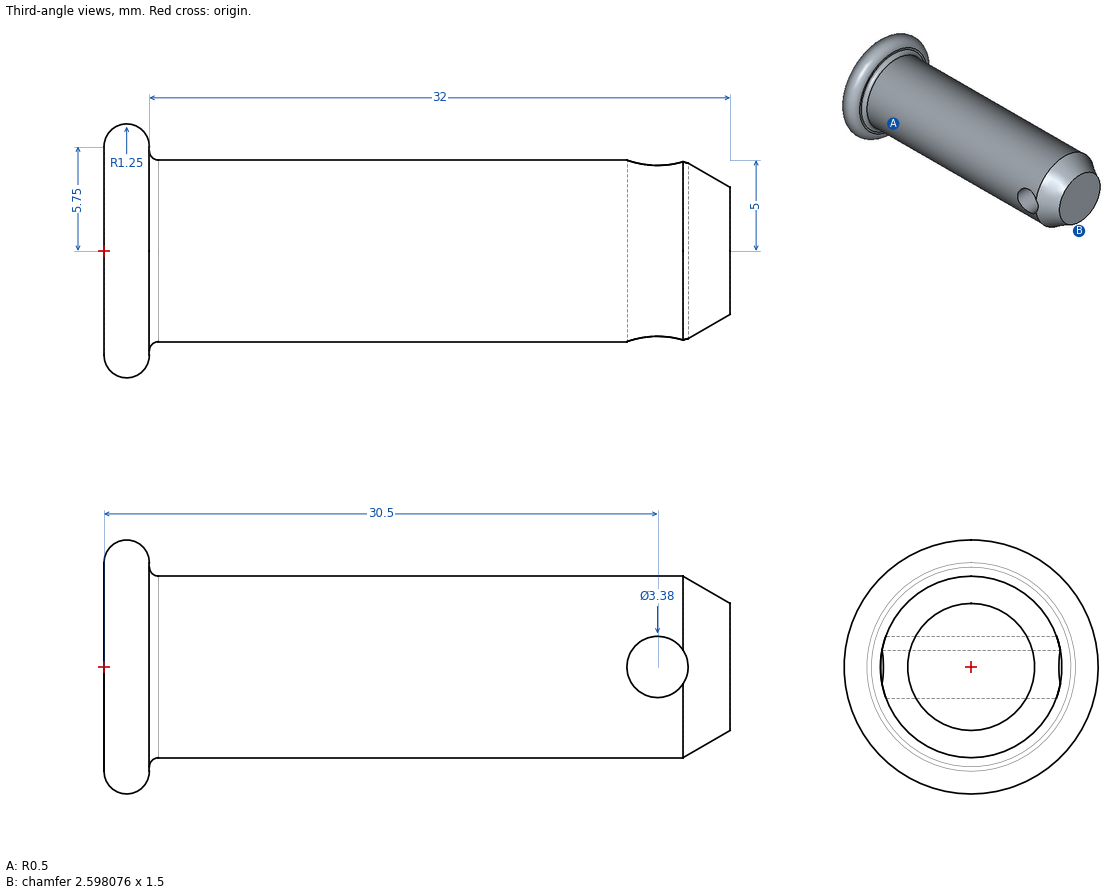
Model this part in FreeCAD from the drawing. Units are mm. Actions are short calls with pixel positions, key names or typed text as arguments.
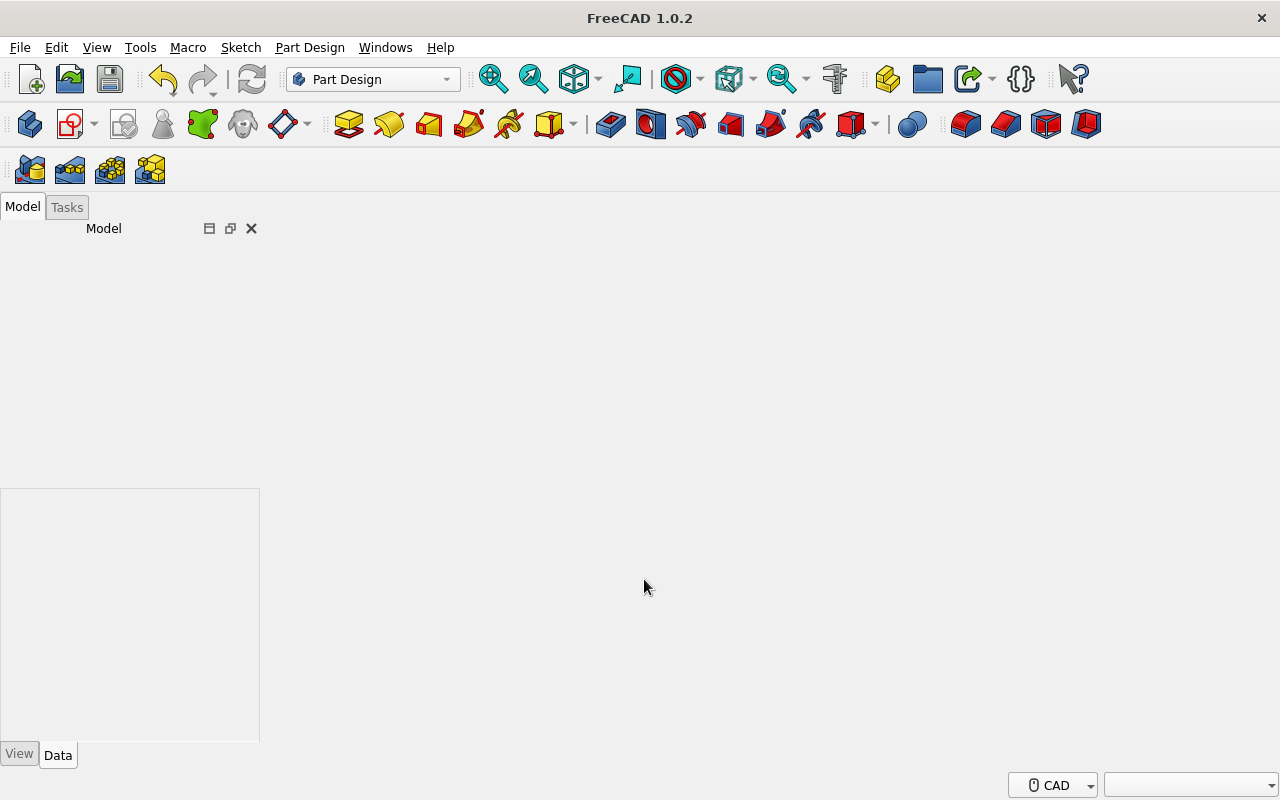
key(ctrl+n)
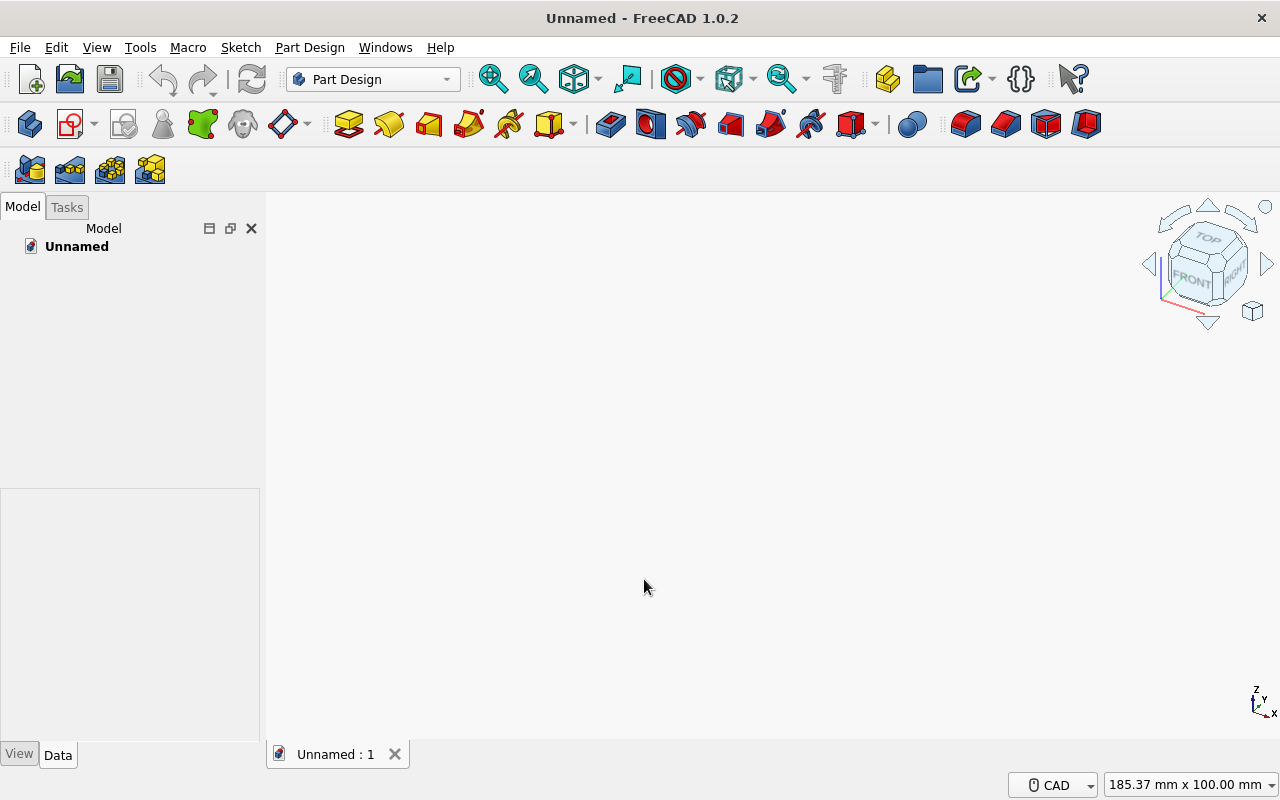
click(70, 124)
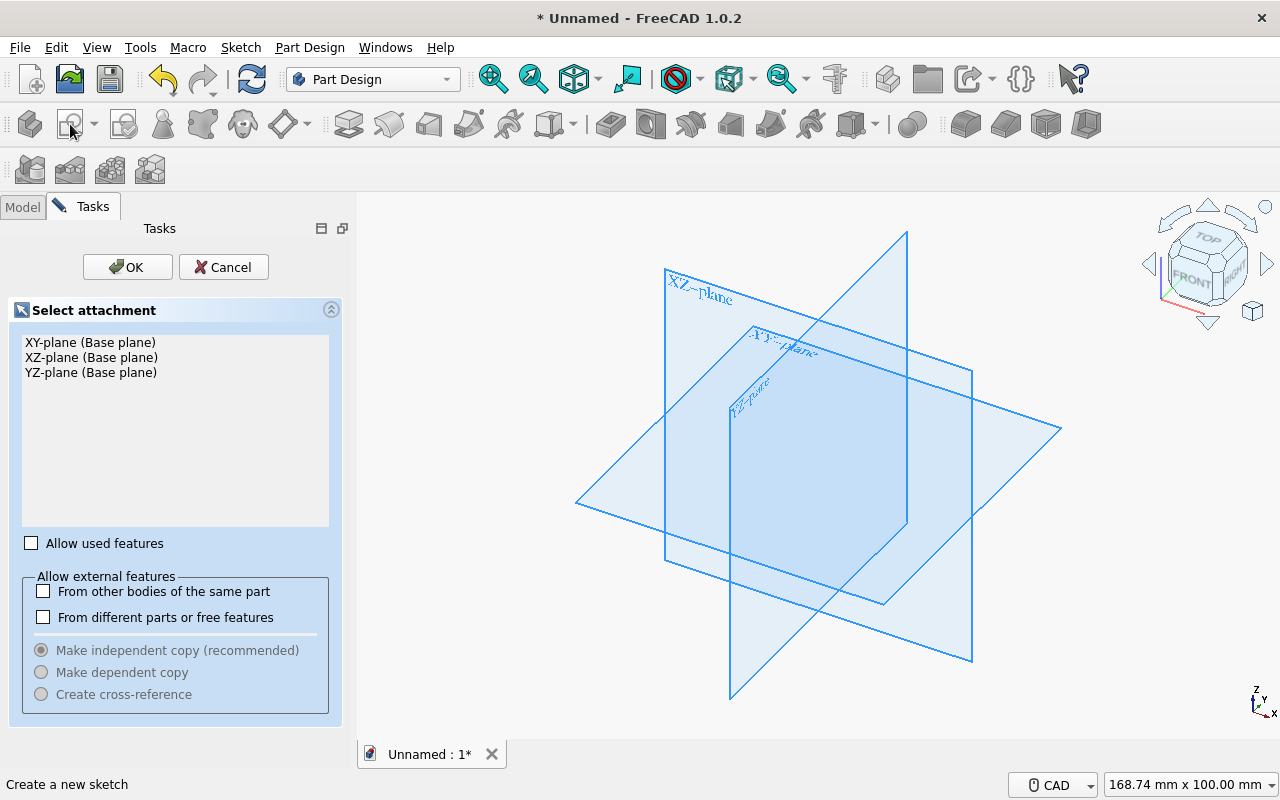
click(82, 342)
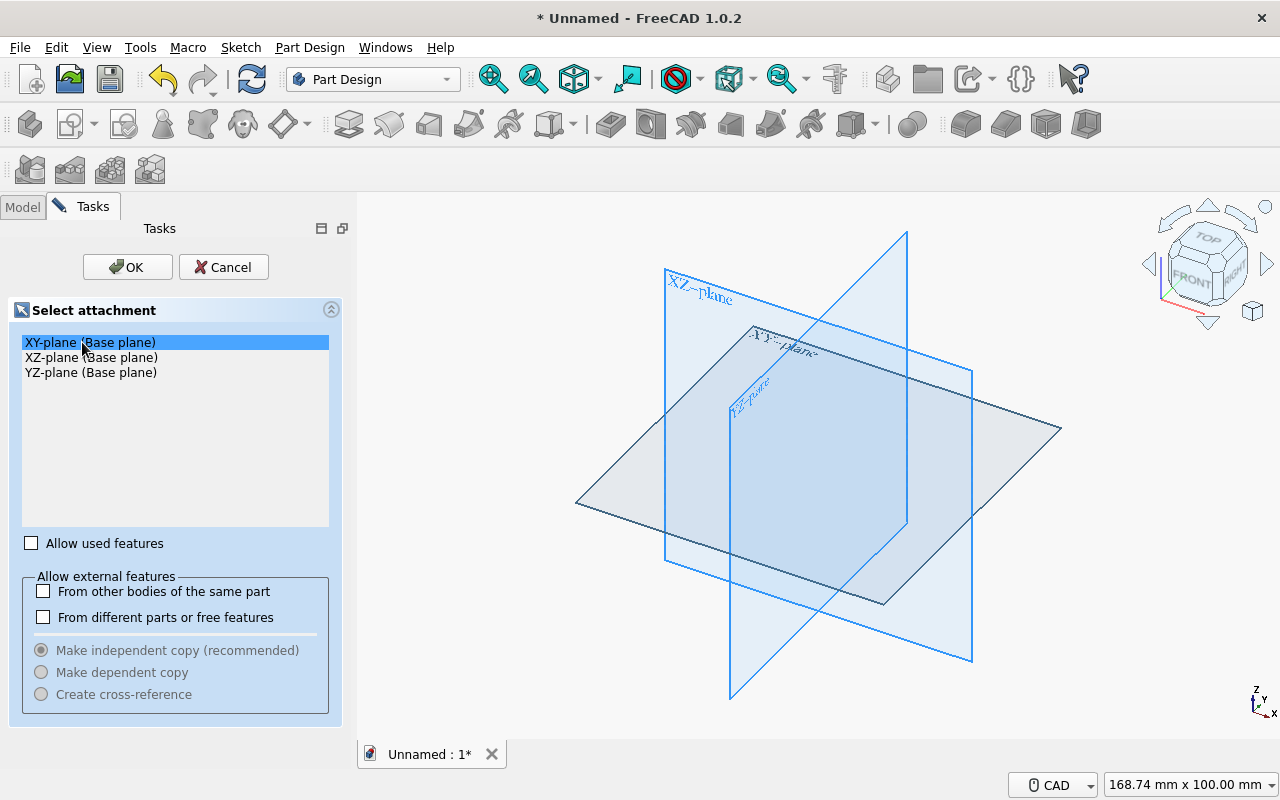
click(128, 267)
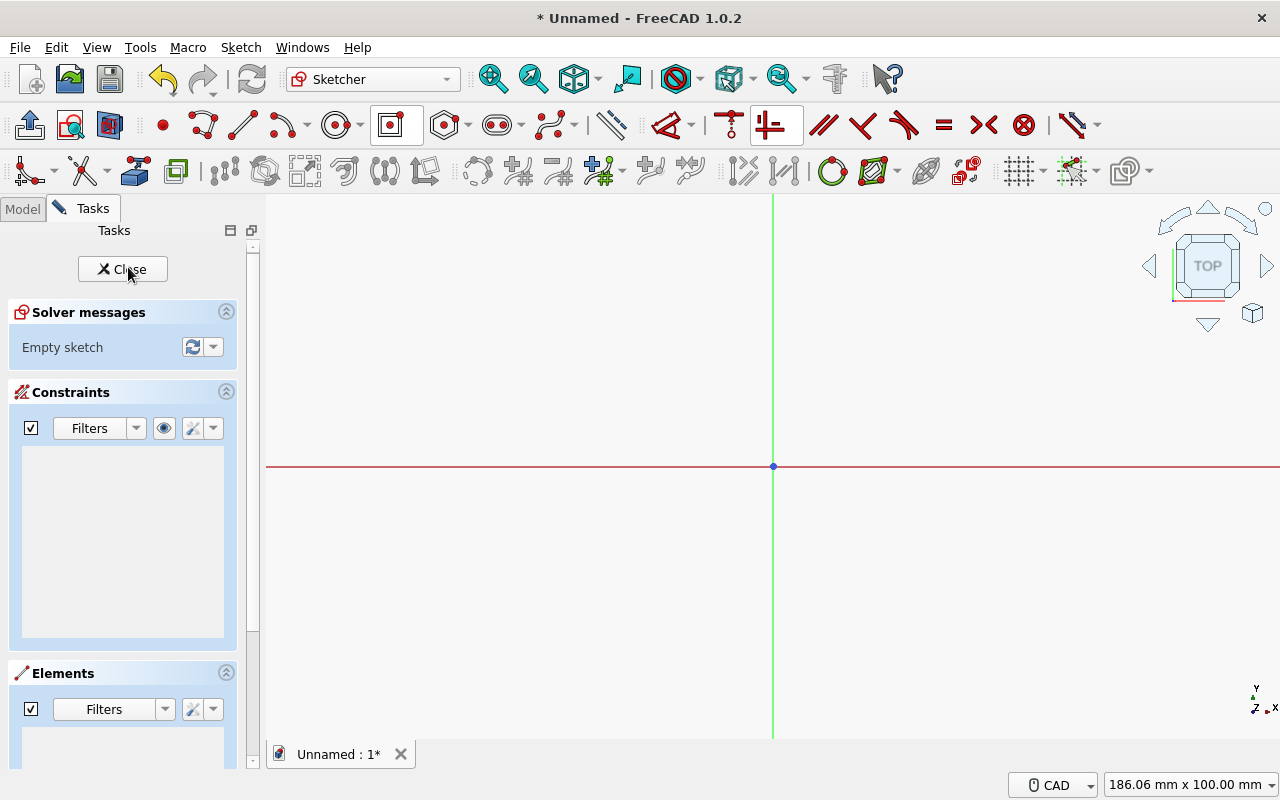
scroll(937, 439, up, 6)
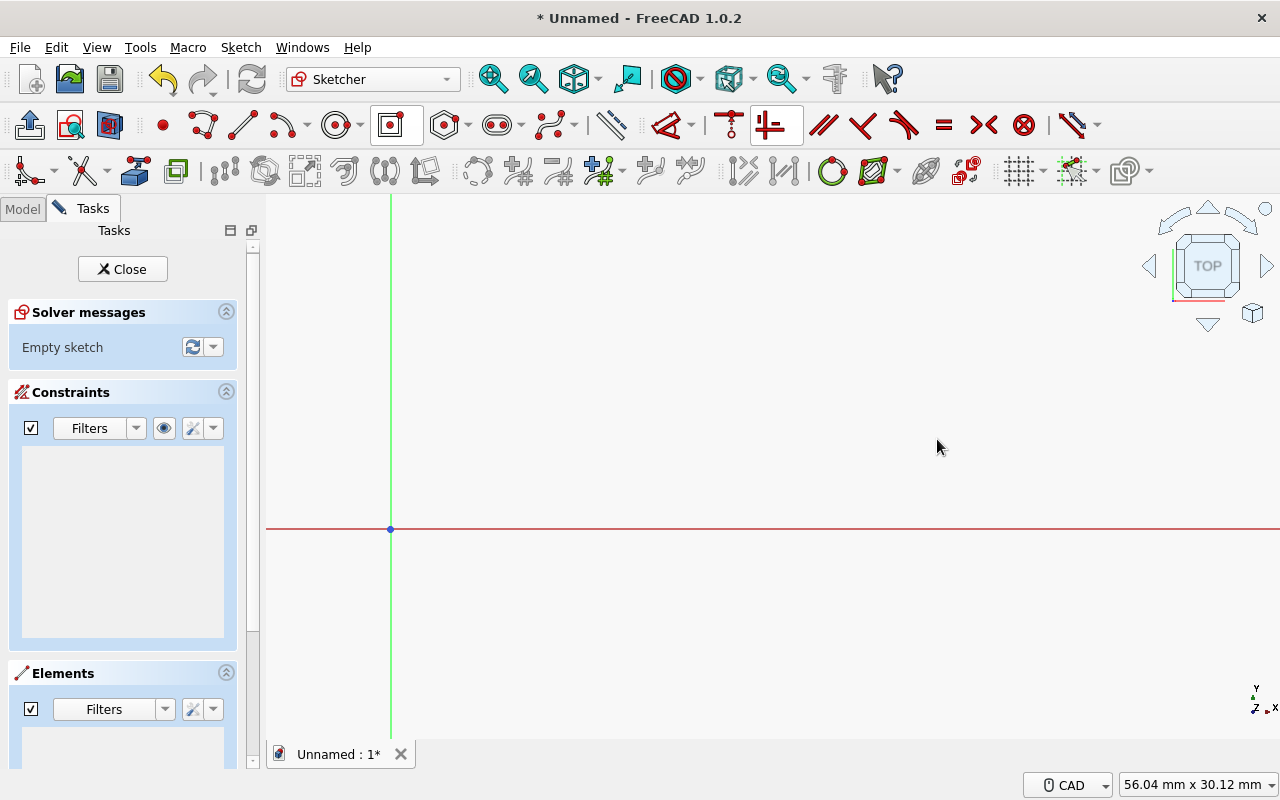
click(204, 126)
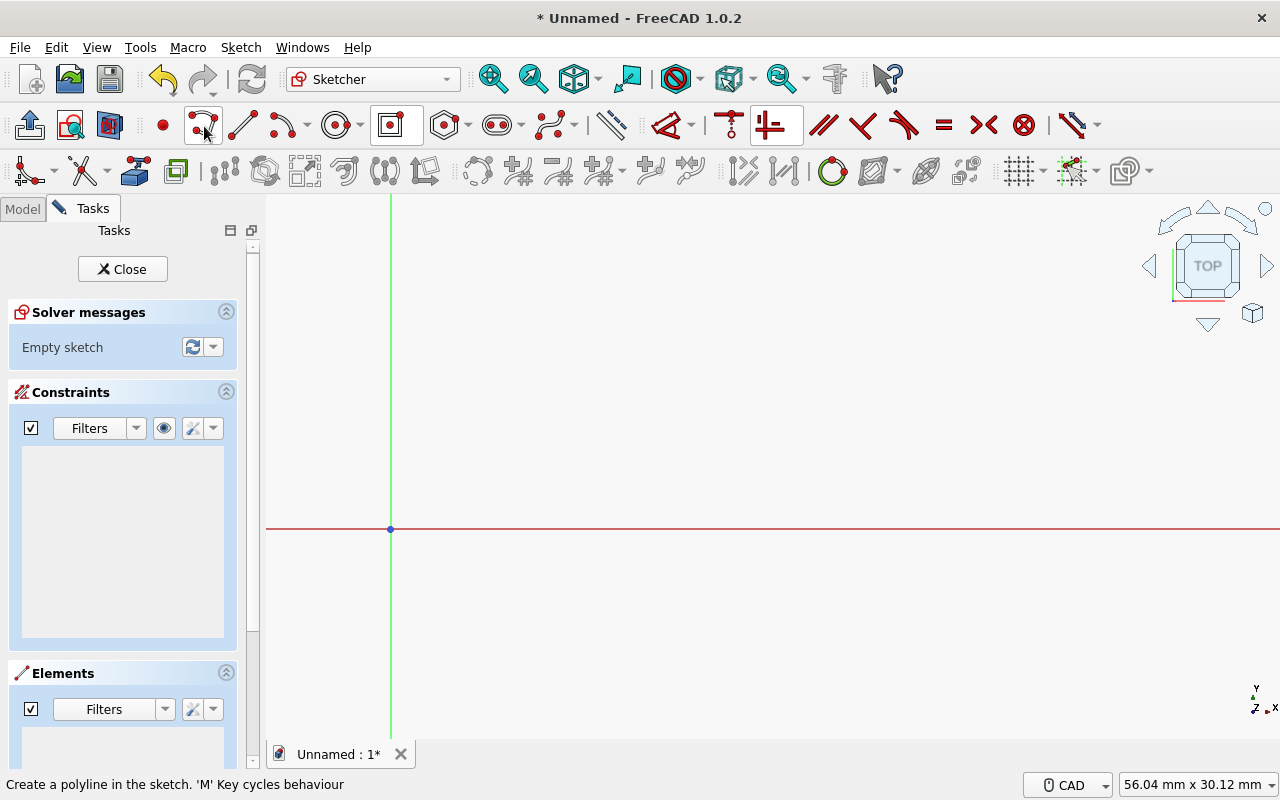
click(391, 425)
click(391, 529)
click(1015, 520)
click(1015, 439)
click(436, 439)
click(436, 425)
right_click(436, 425)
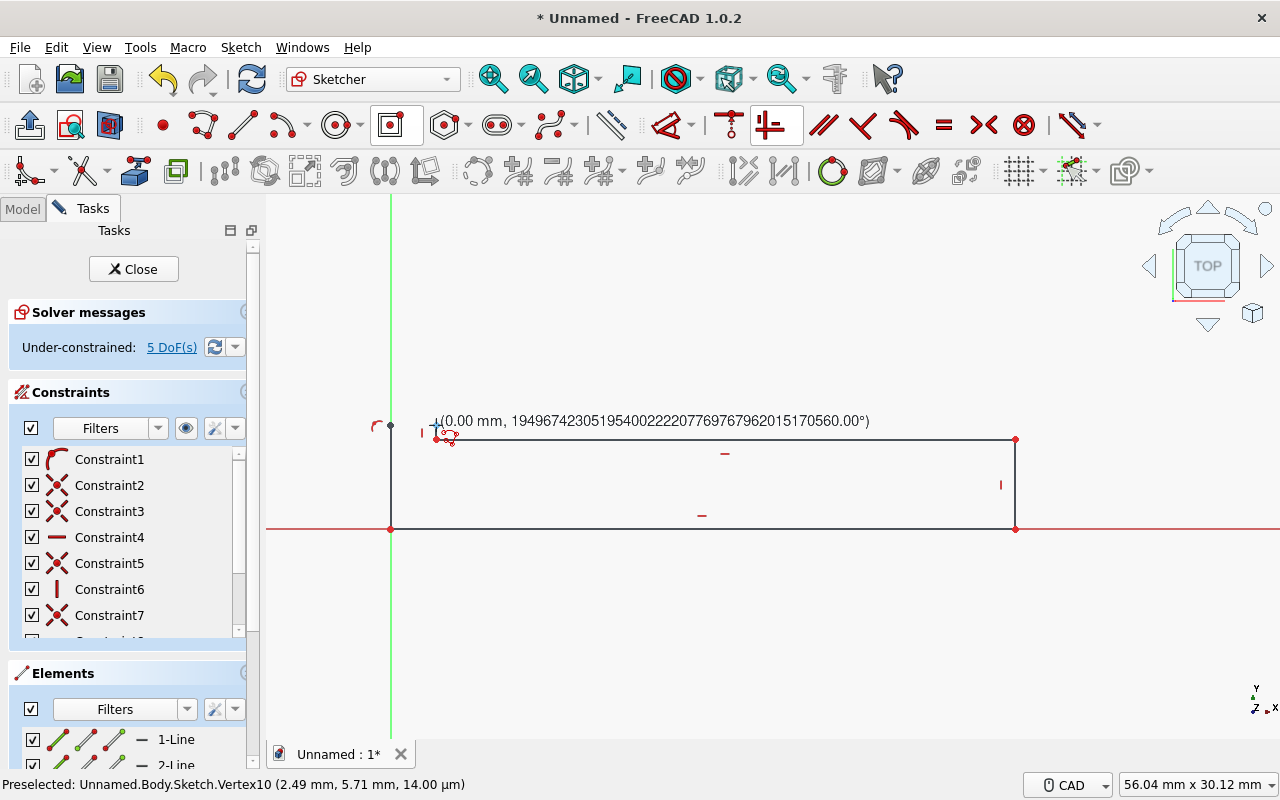
key(g)
key(3)
key(a)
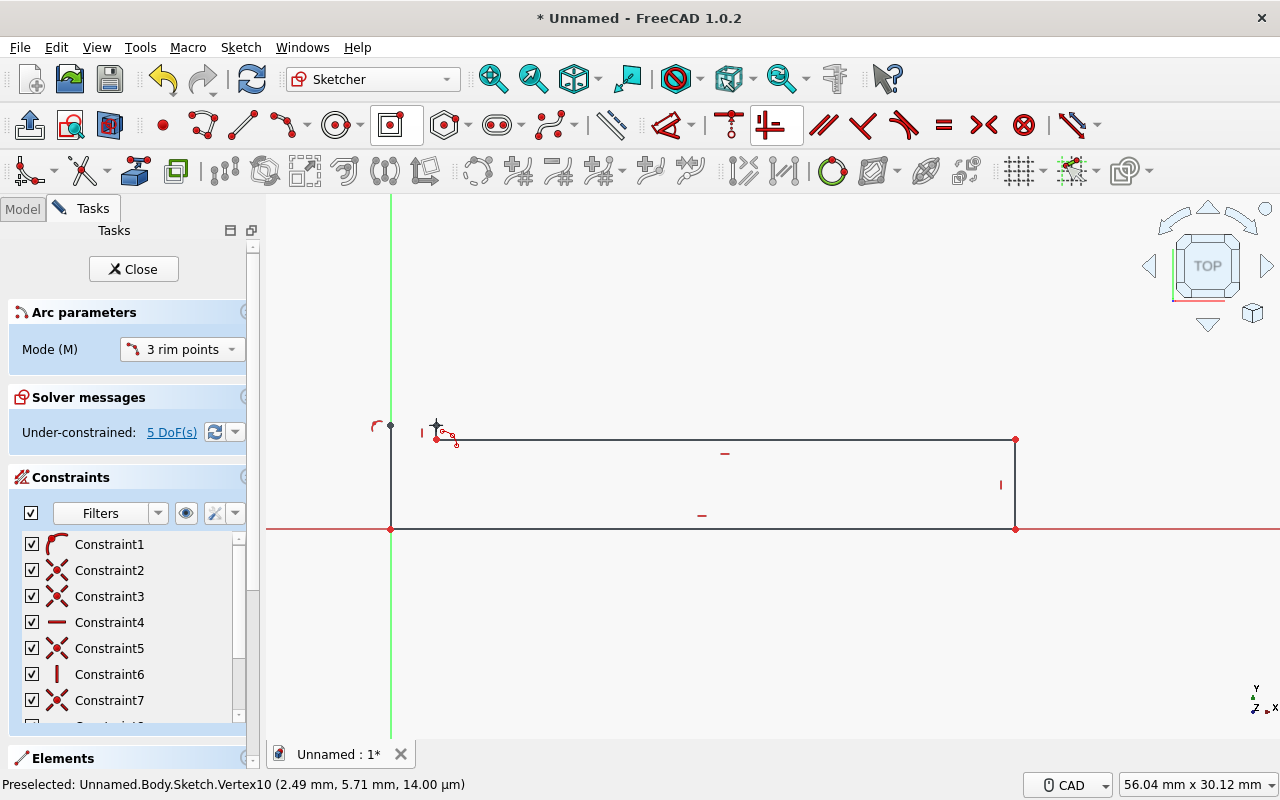
scroll(436, 425, up, 5)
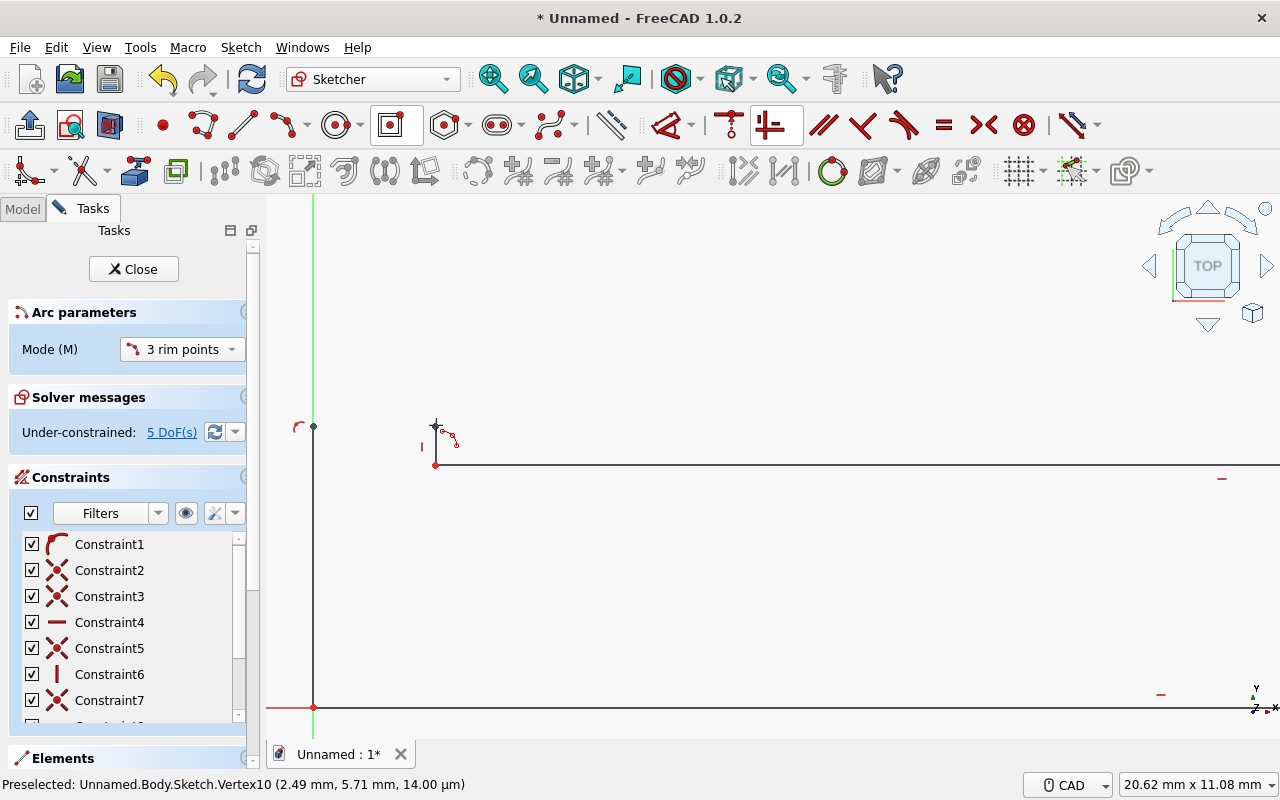
click(436, 427)
click(313, 427)
click(375, 363)
key(Escape)